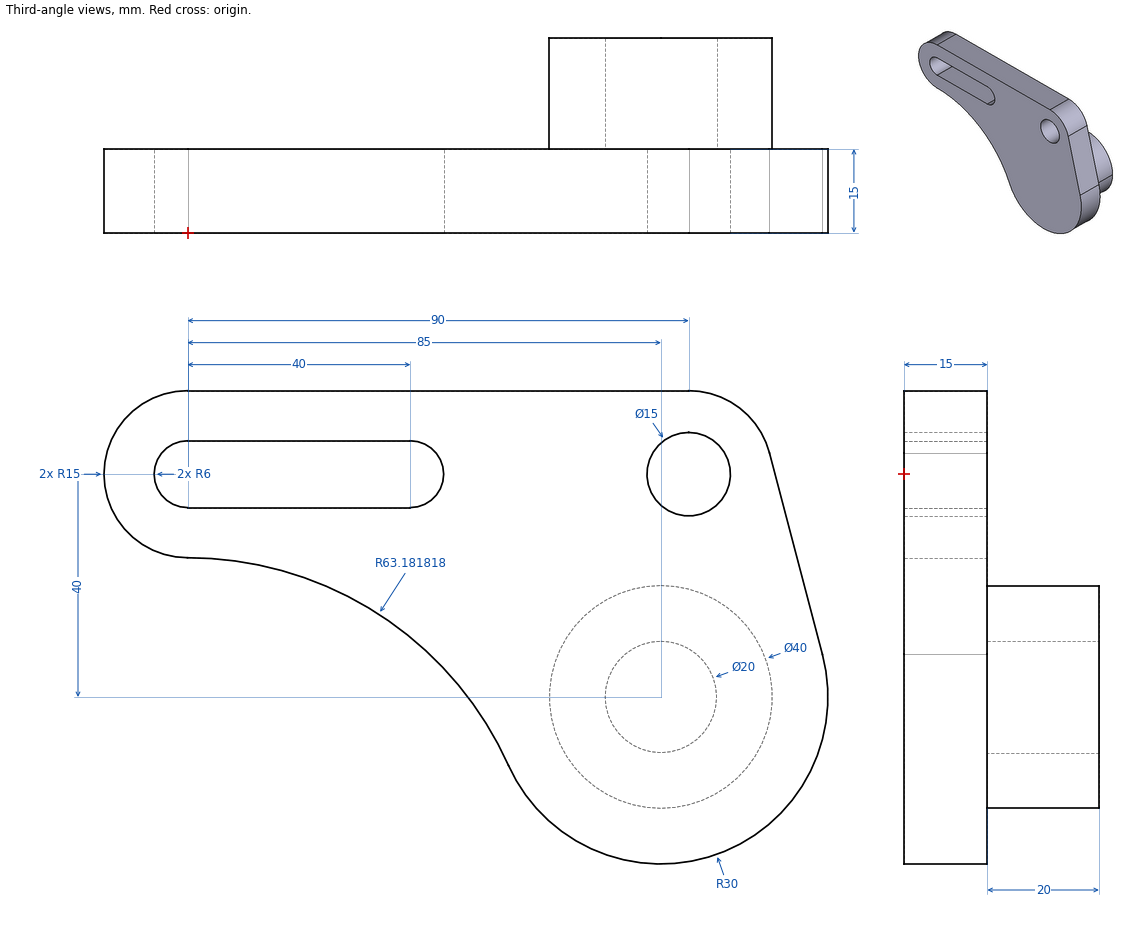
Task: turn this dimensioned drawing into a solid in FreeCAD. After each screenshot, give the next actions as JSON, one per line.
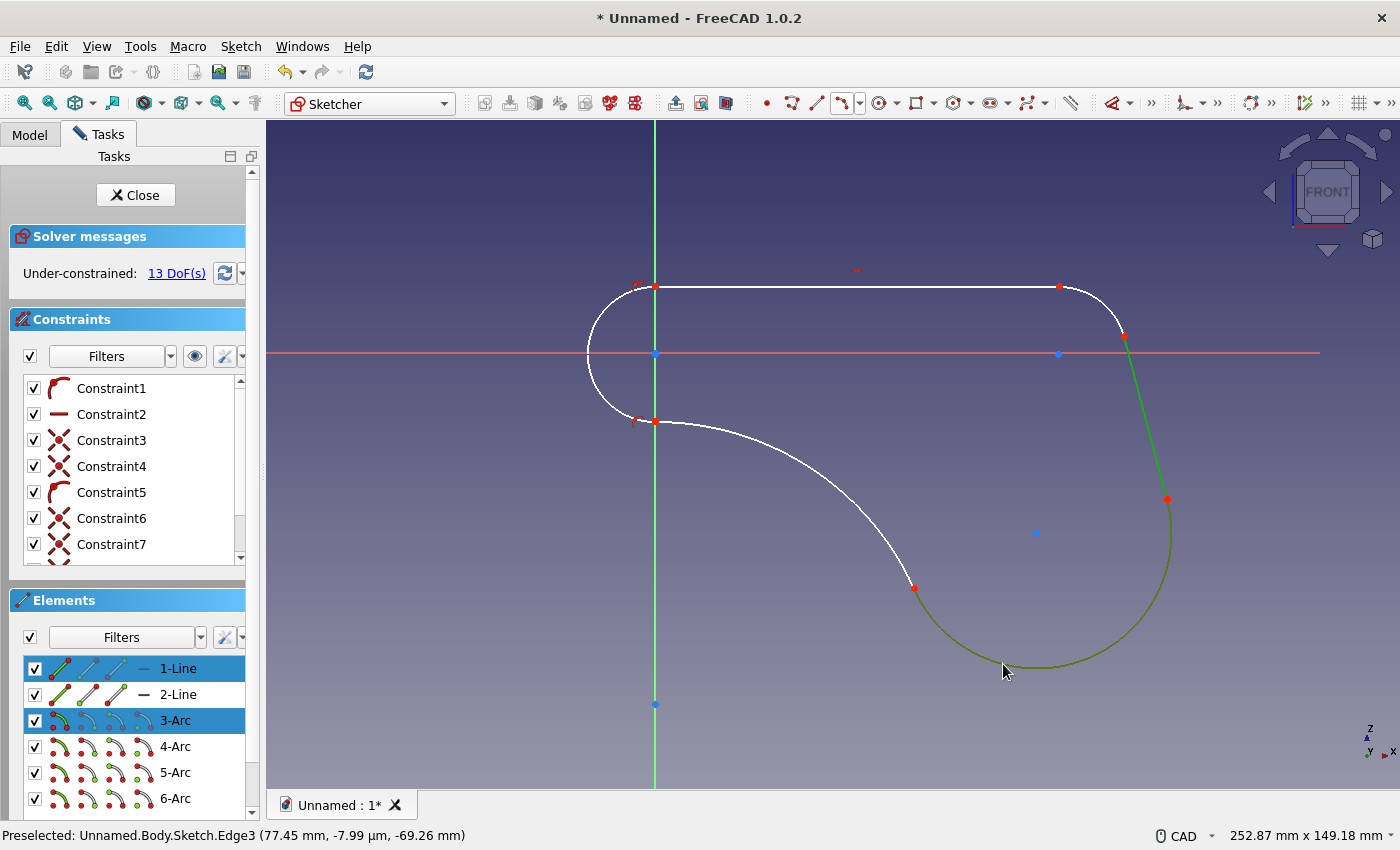
{"action": "key", "text": "t"}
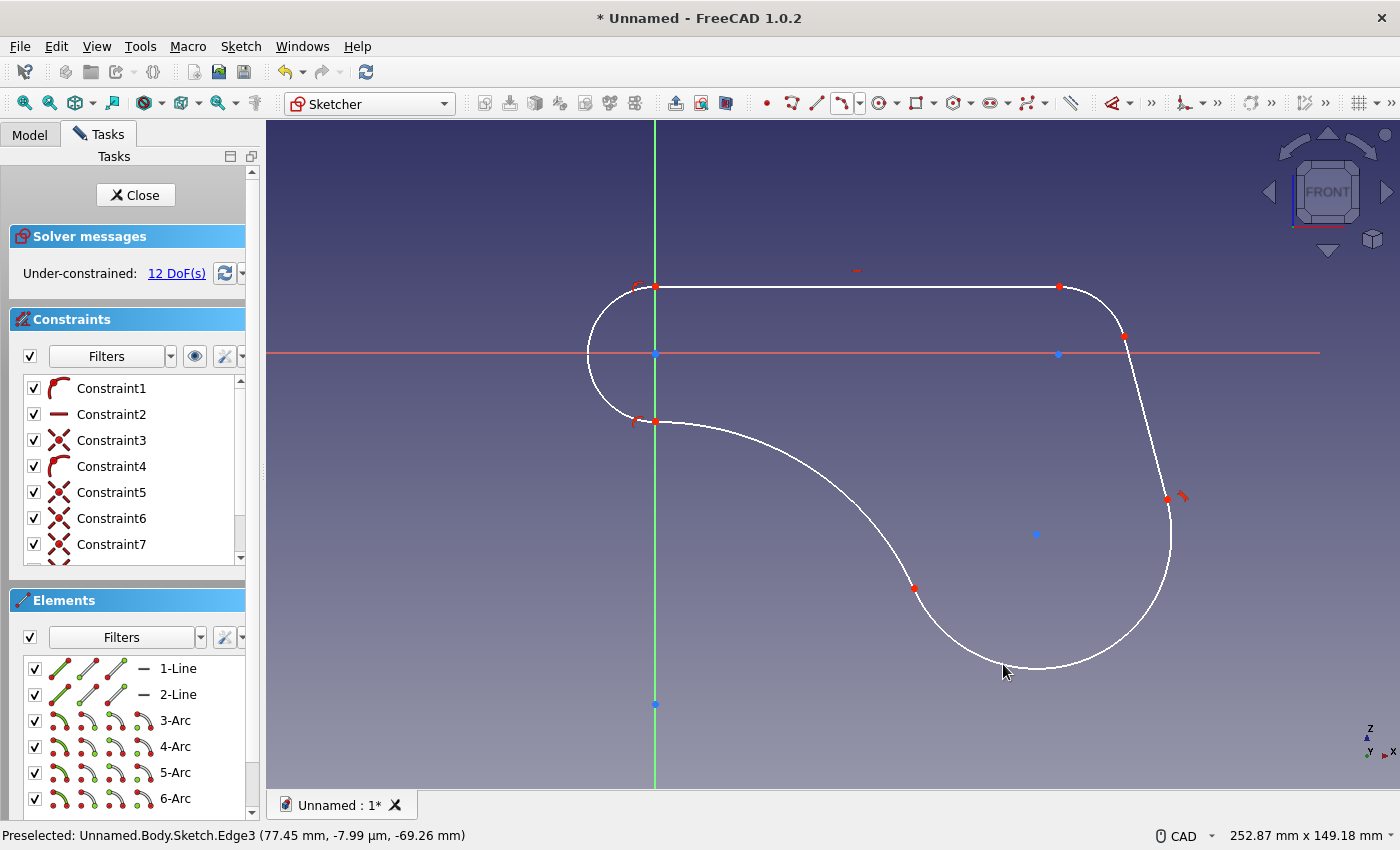
{"action": "left_click", "coordinate": [1137, 386]}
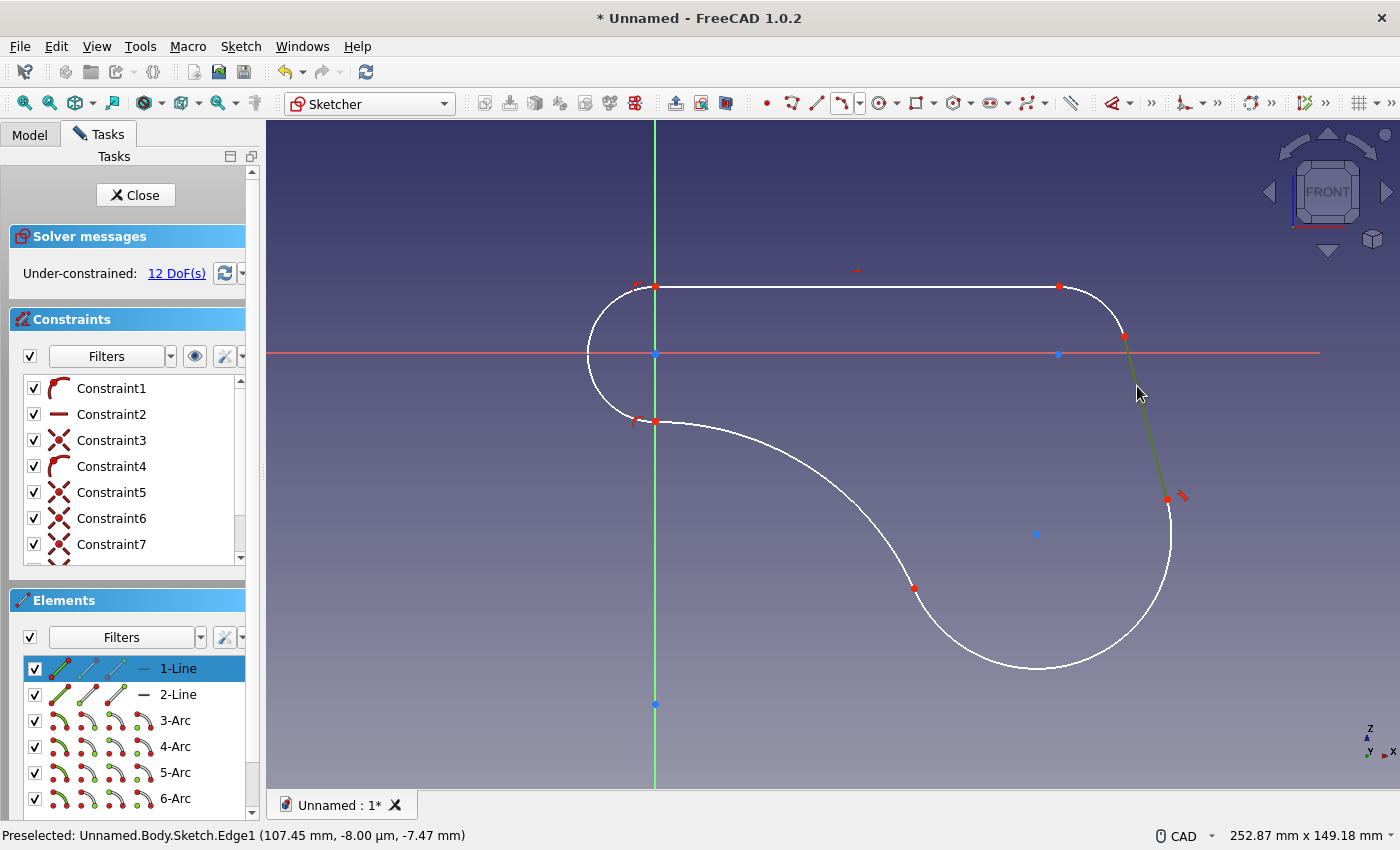
{"action": "left_click", "coordinate": [1112, 313]}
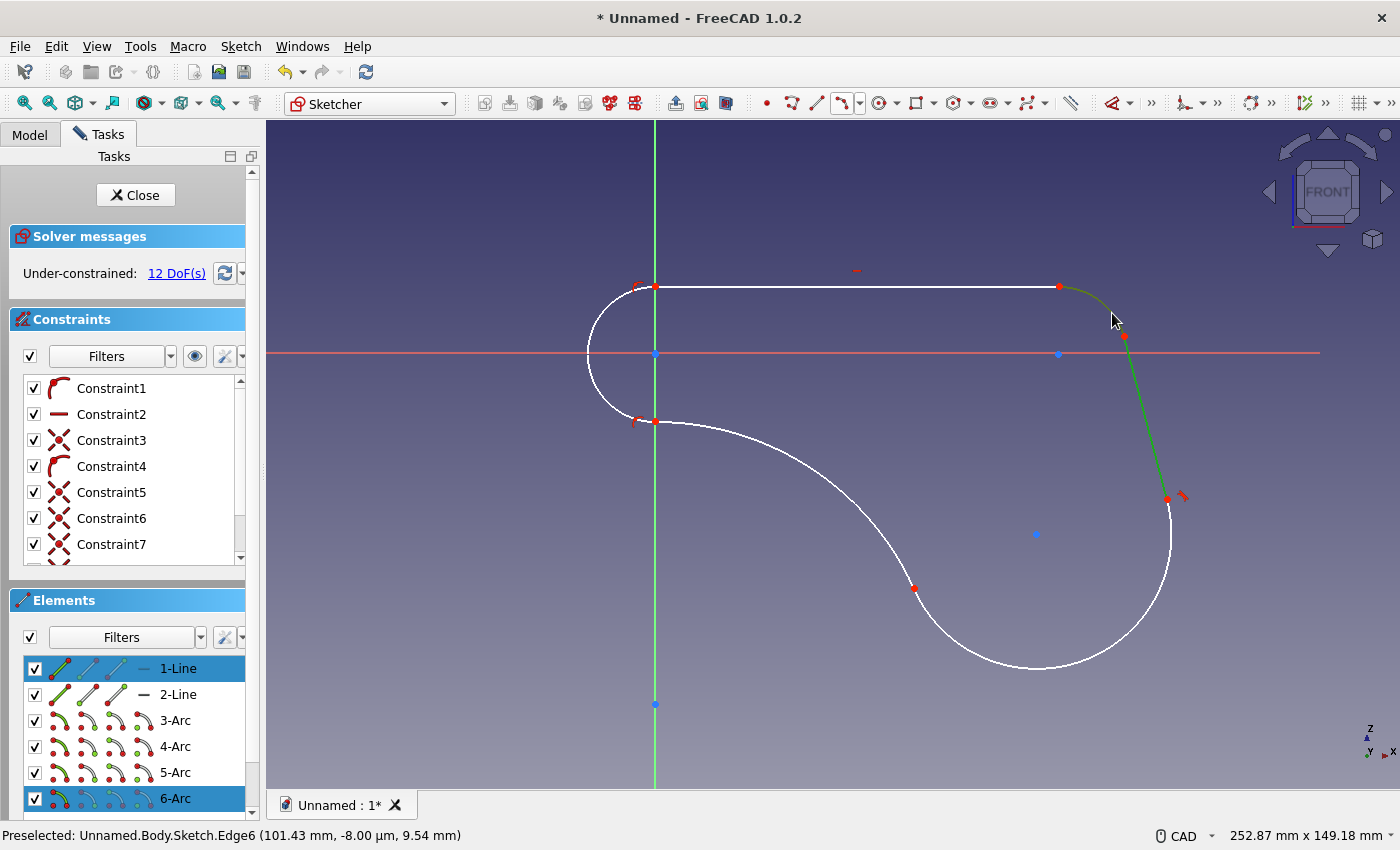
{"action": "key", "text": "t"}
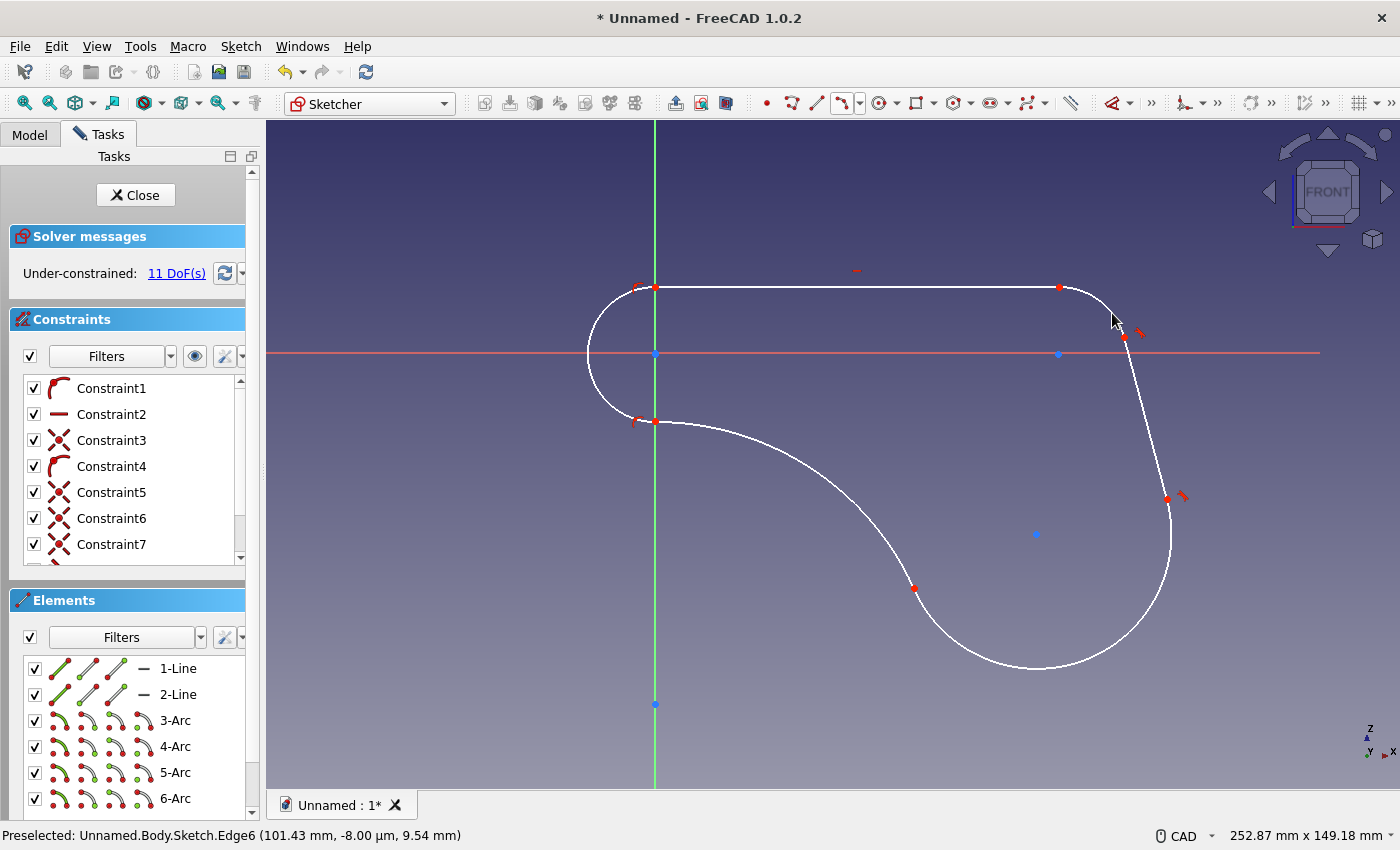
{"action": "left_click", "coordinate": [776, 287]}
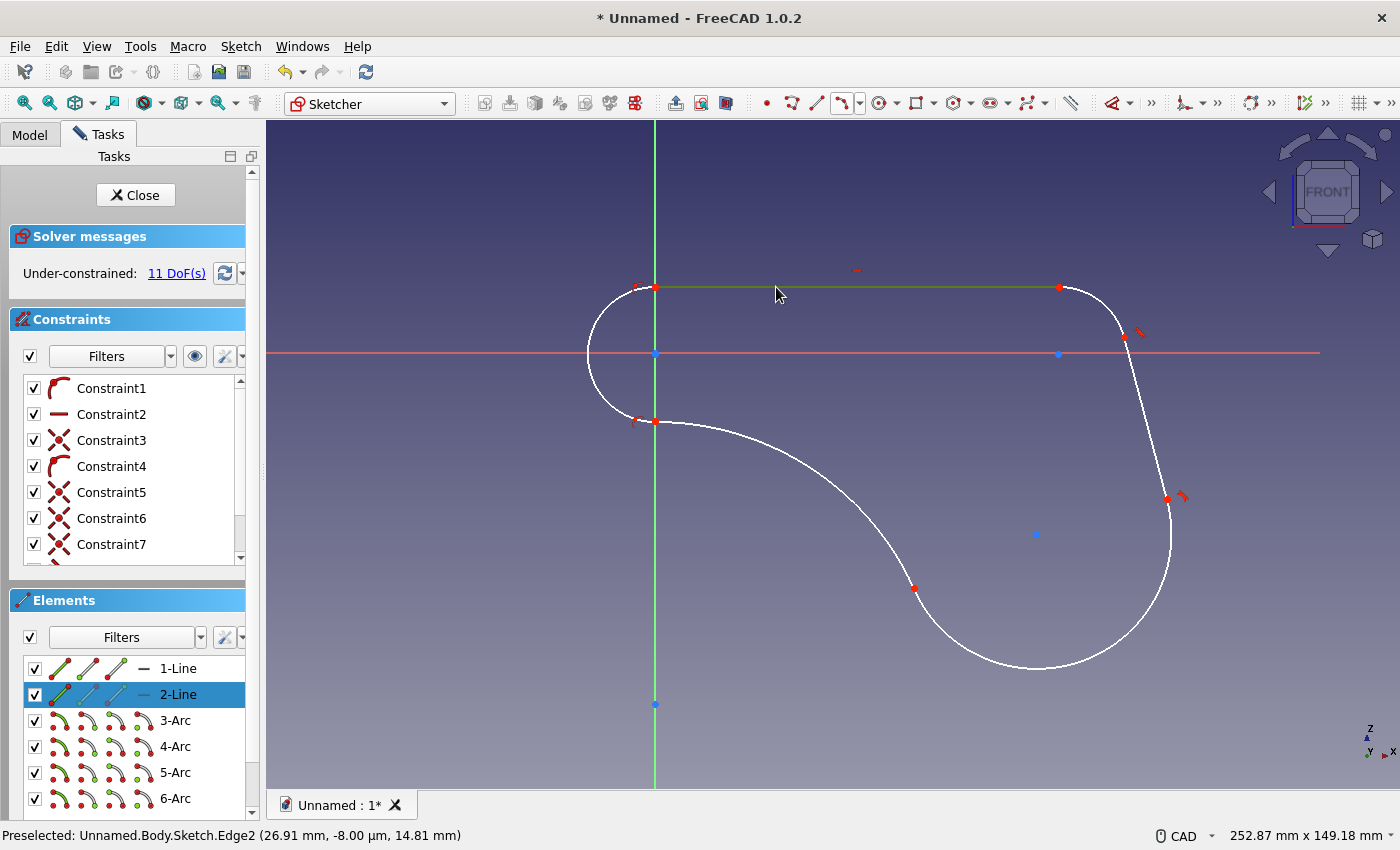
{"action": "left_click", "coordinate": [601, 315]}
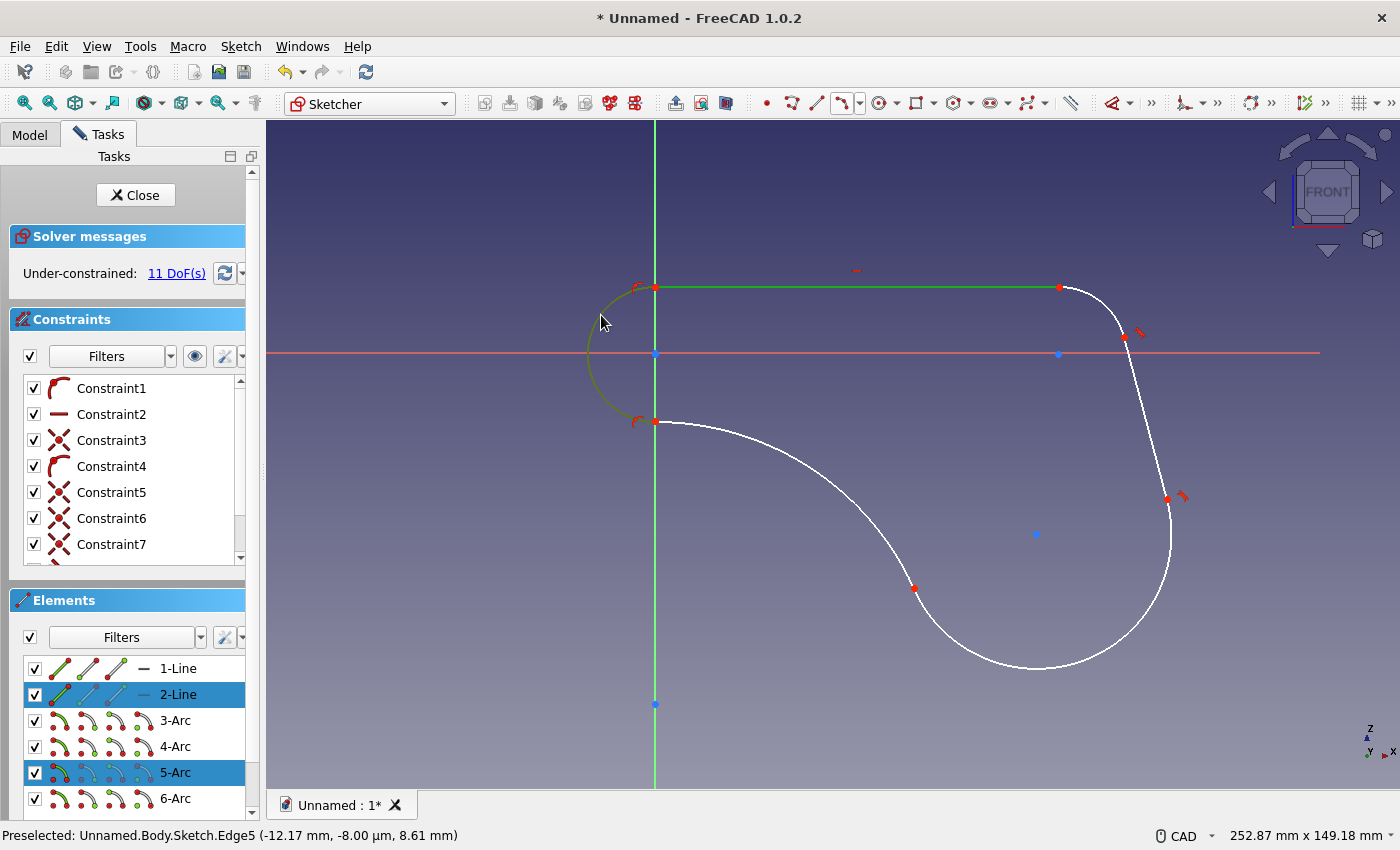
{"action": "key", "text": "t"}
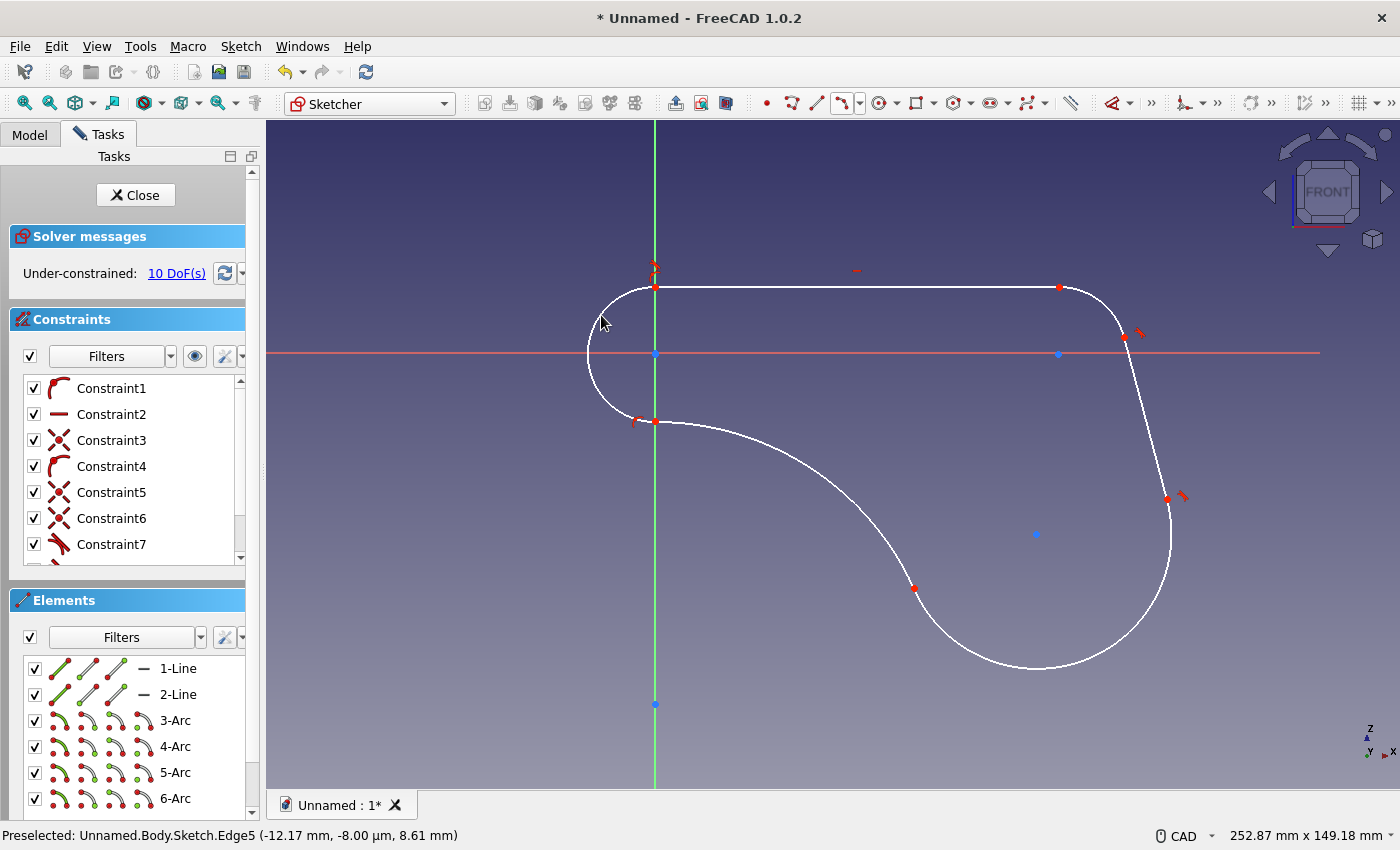
{"action": "left_click", "coordinate": [776, 287]}